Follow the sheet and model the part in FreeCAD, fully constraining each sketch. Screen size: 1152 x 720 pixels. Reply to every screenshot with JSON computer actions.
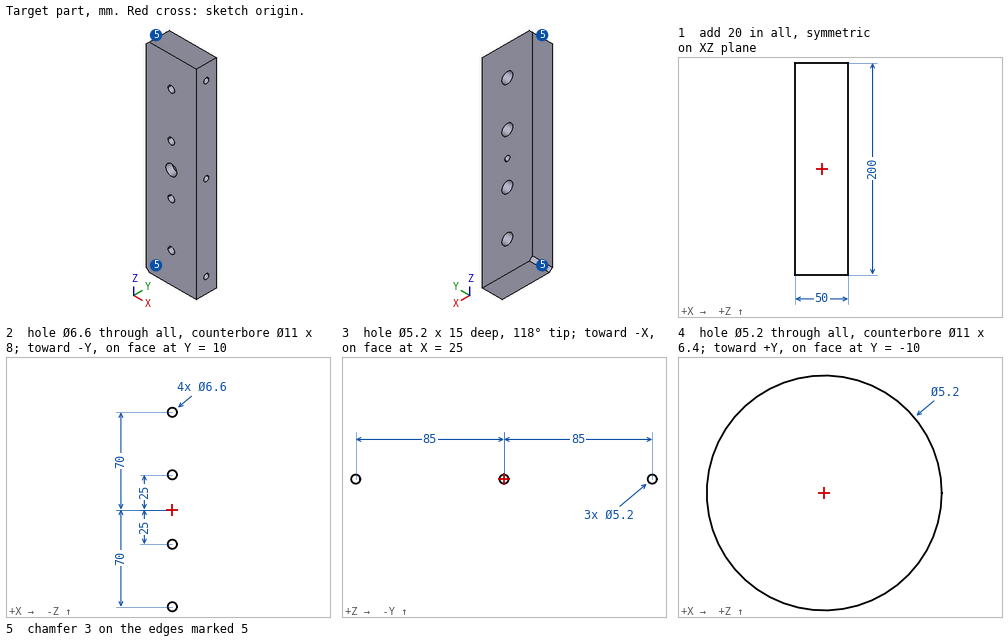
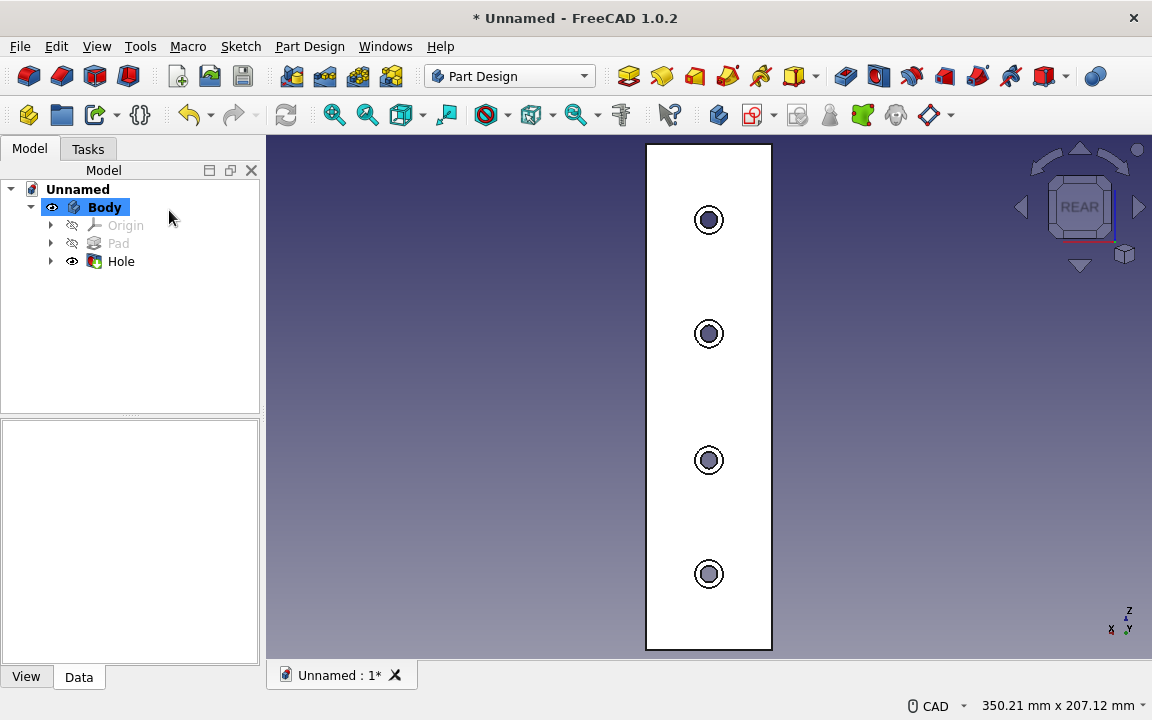
{"action": "key", "text": "0"}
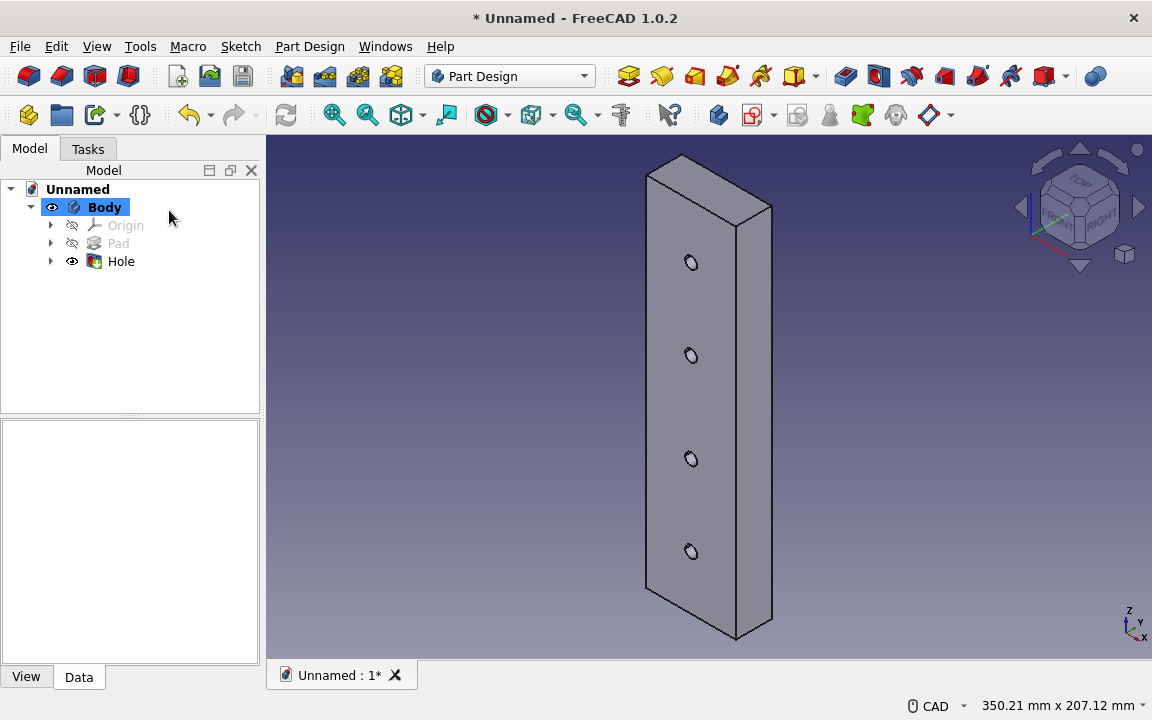
{"action": "left_click", "coordinate": [754, 245]}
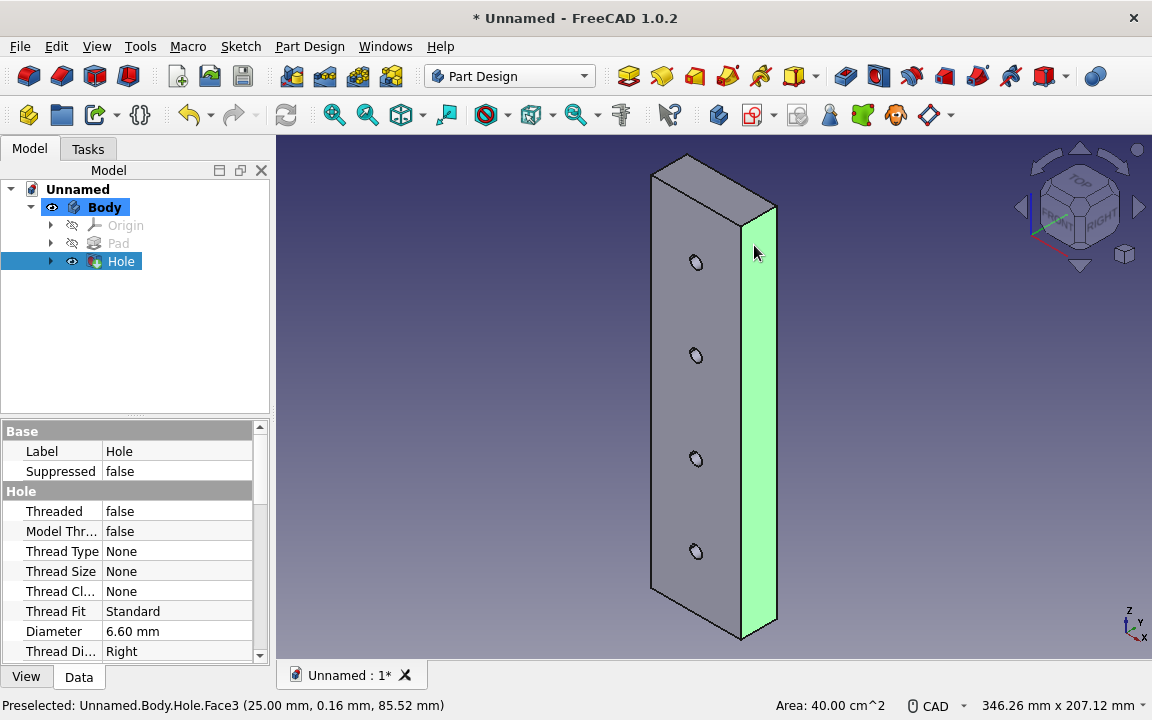
{"action": "left_click", "coordinate": [752, 116]}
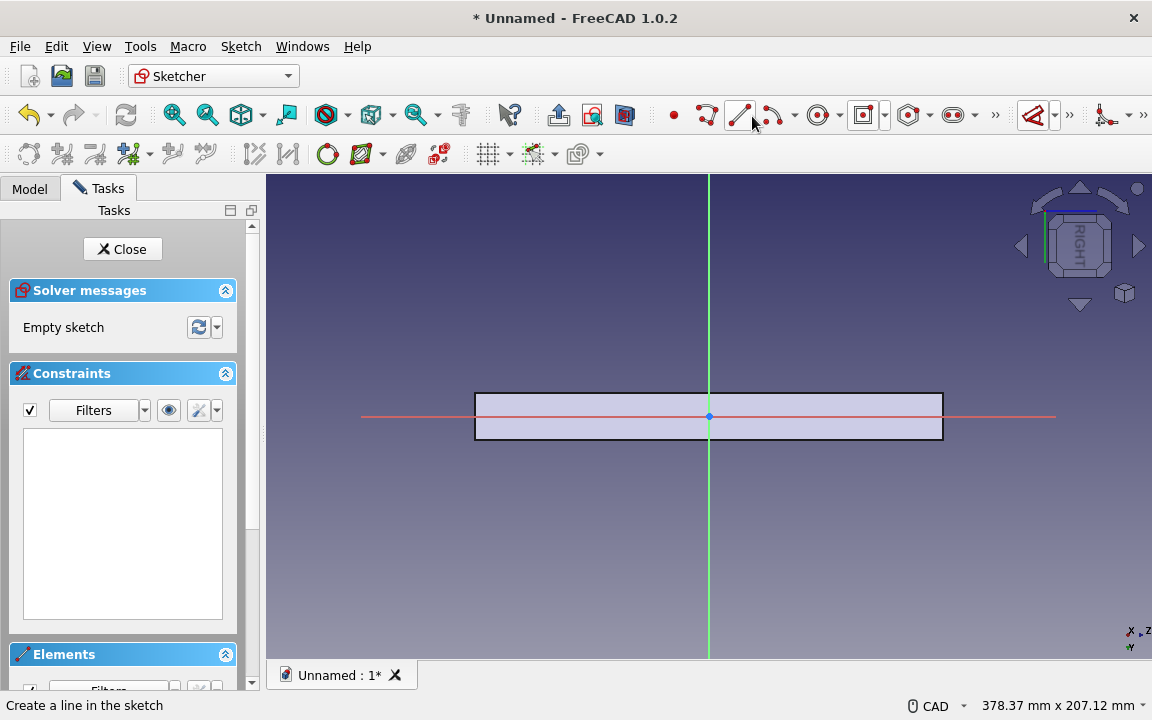
{"action": "left_click", "coordinate": [818, 116]}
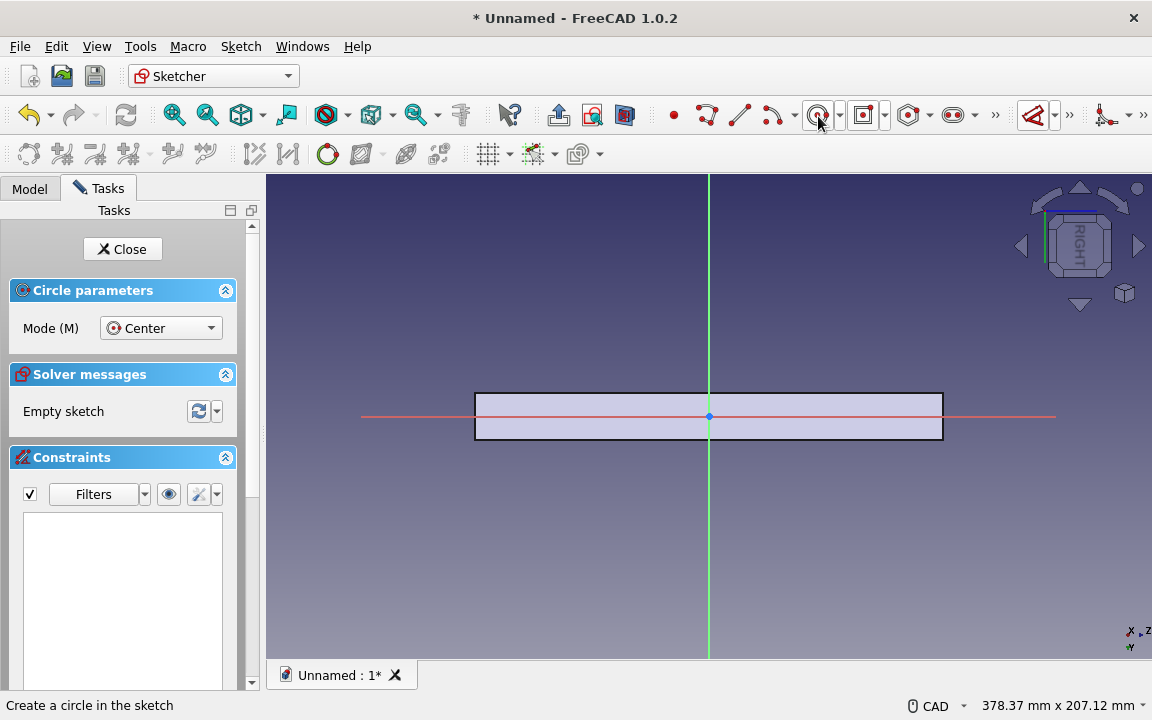
{"action": "scroll", "coordinate": [908, 417], "scroll_direction": "up", "scroll_amount": 7}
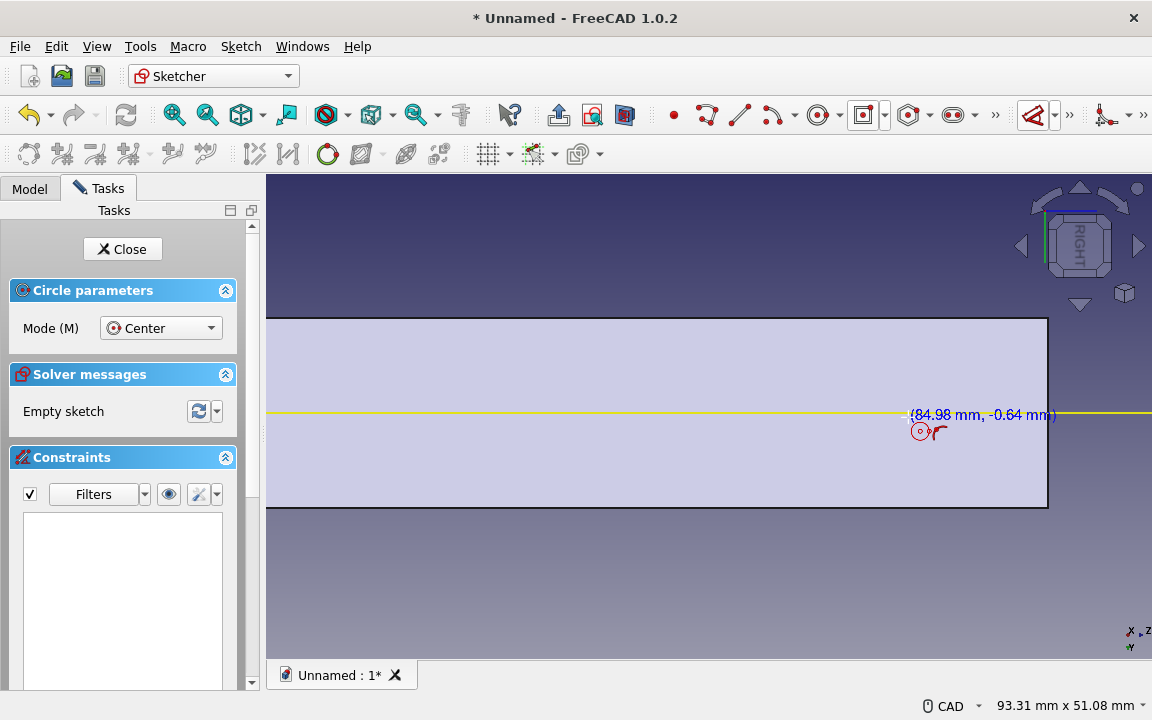
{"action": "scroll", "coordinate": [874, 418], "scroll_direction": "down", "scroll_amount": 6}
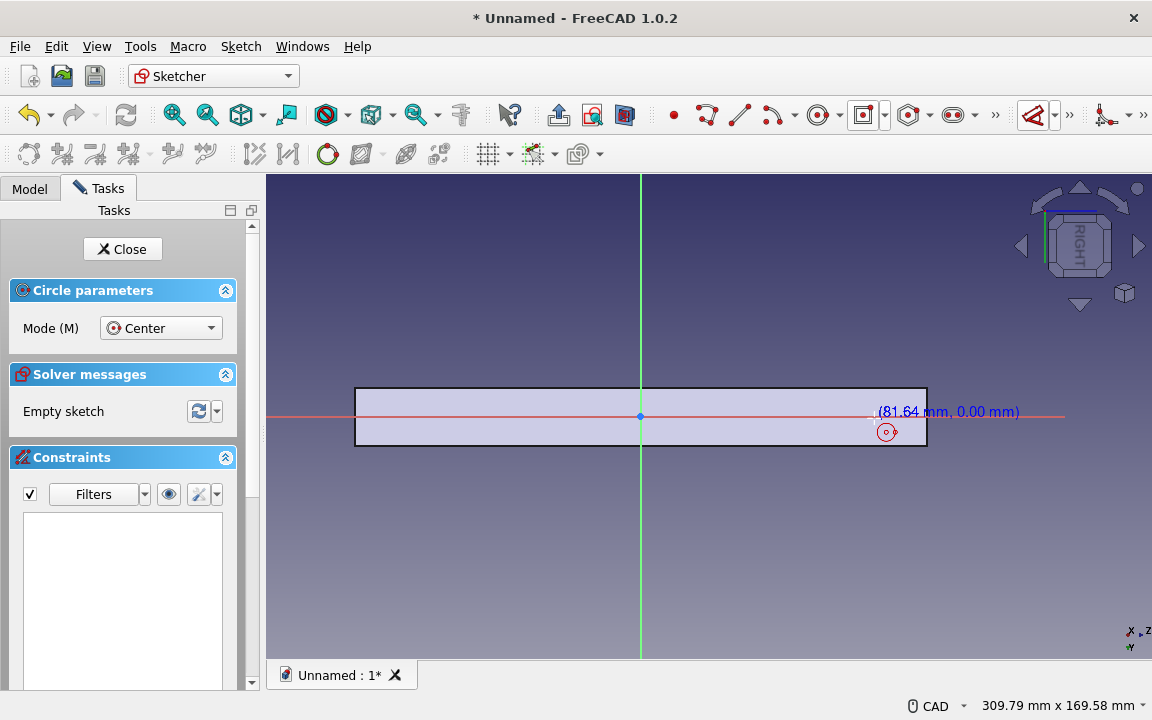
{"action": "left_click", "coordinate": [884, 417]}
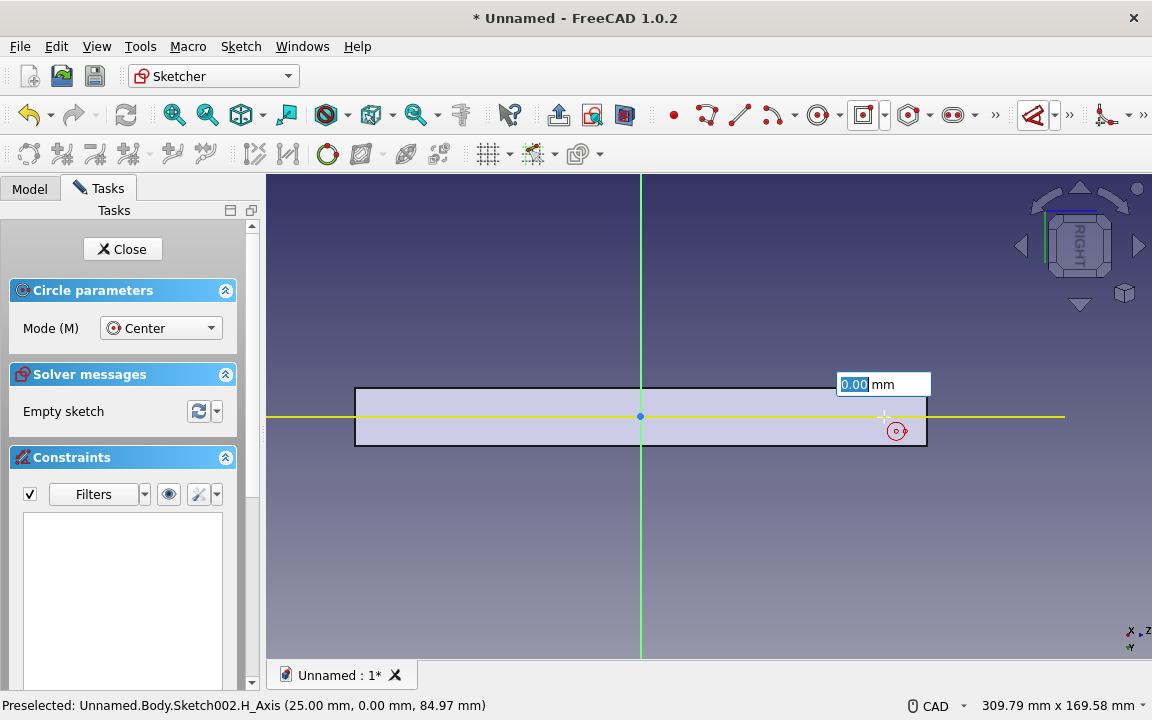
{"action": "scroll", "coordinate": [882, 424], "scroll_direction": "up", "scroll_amount": 5}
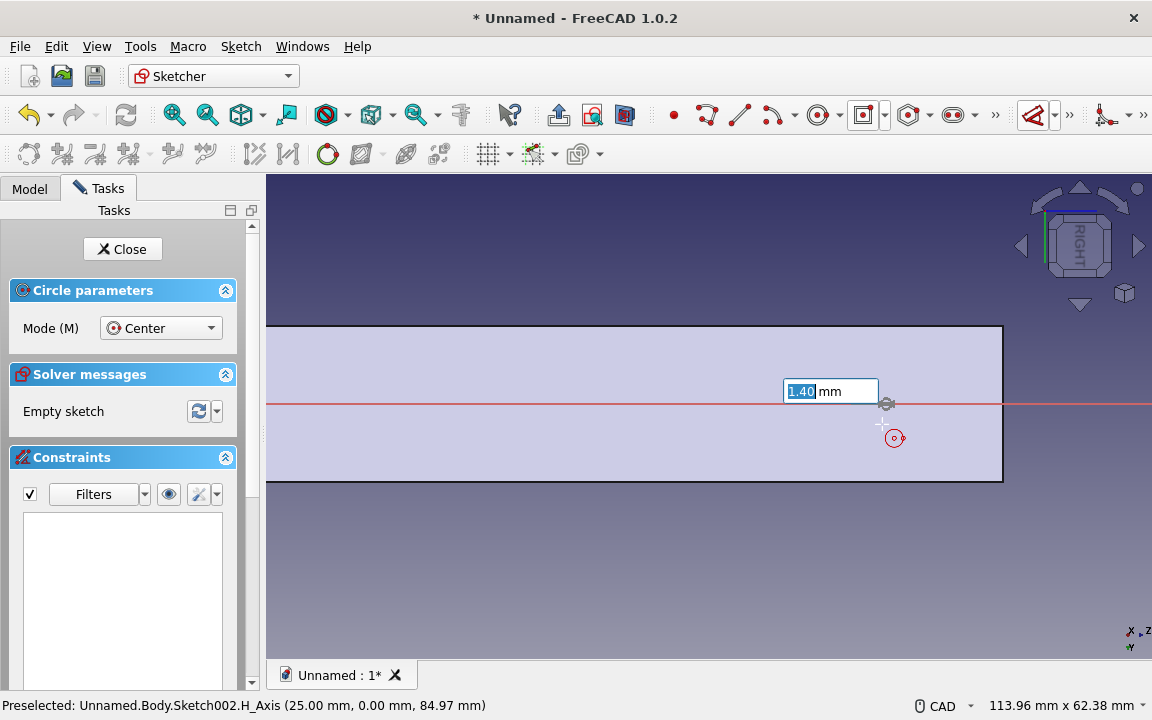
{"action": "left_click", "coordinate": [880, 423]}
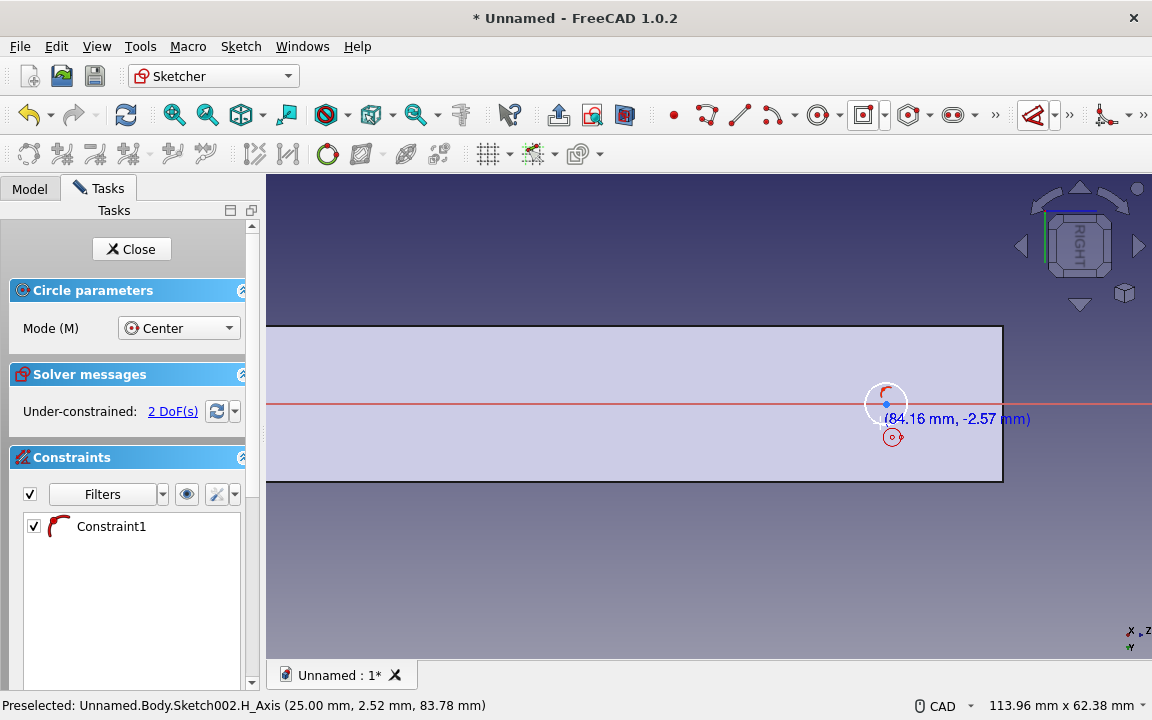
{"action": "scroll", "coordinate": [882, 424], "scroll_direction": "down", "scroll_amount": 5}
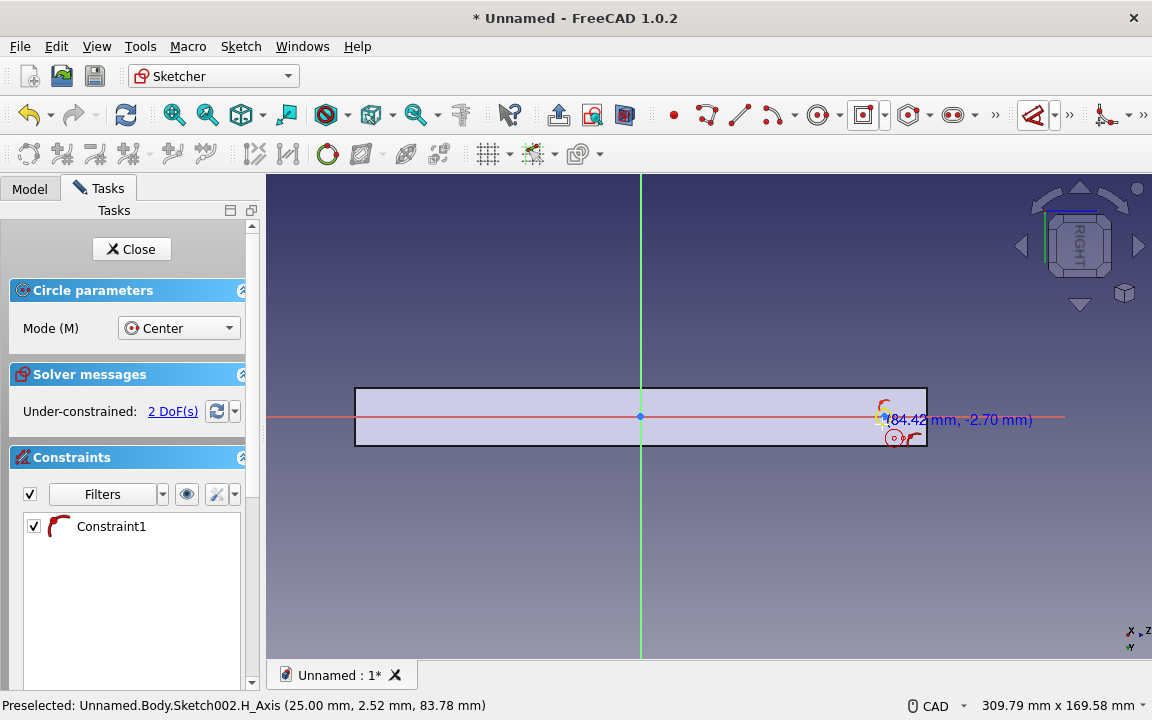
{"action": "scroll", "coordinate": [641, 417], "scroll_direction": "up", "scroll_amount": 6}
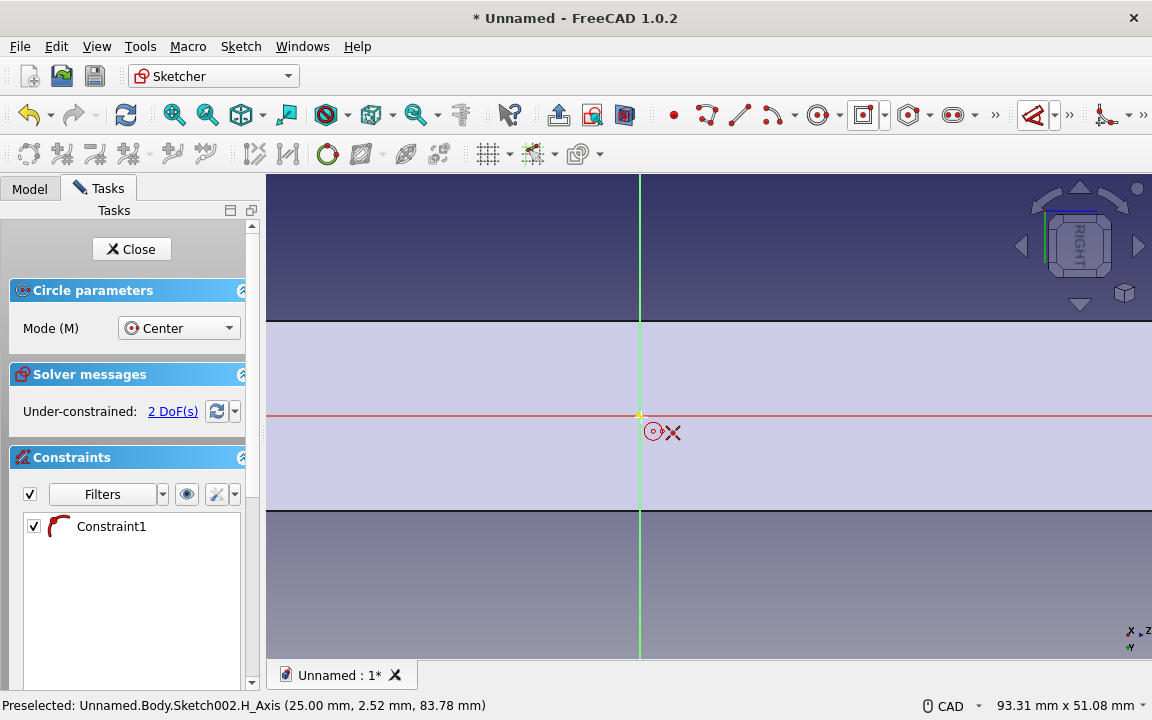
{"action": "scroll", "coordinate": [641, 417], "scroll_direction": "down", "scroll_amount": 6}